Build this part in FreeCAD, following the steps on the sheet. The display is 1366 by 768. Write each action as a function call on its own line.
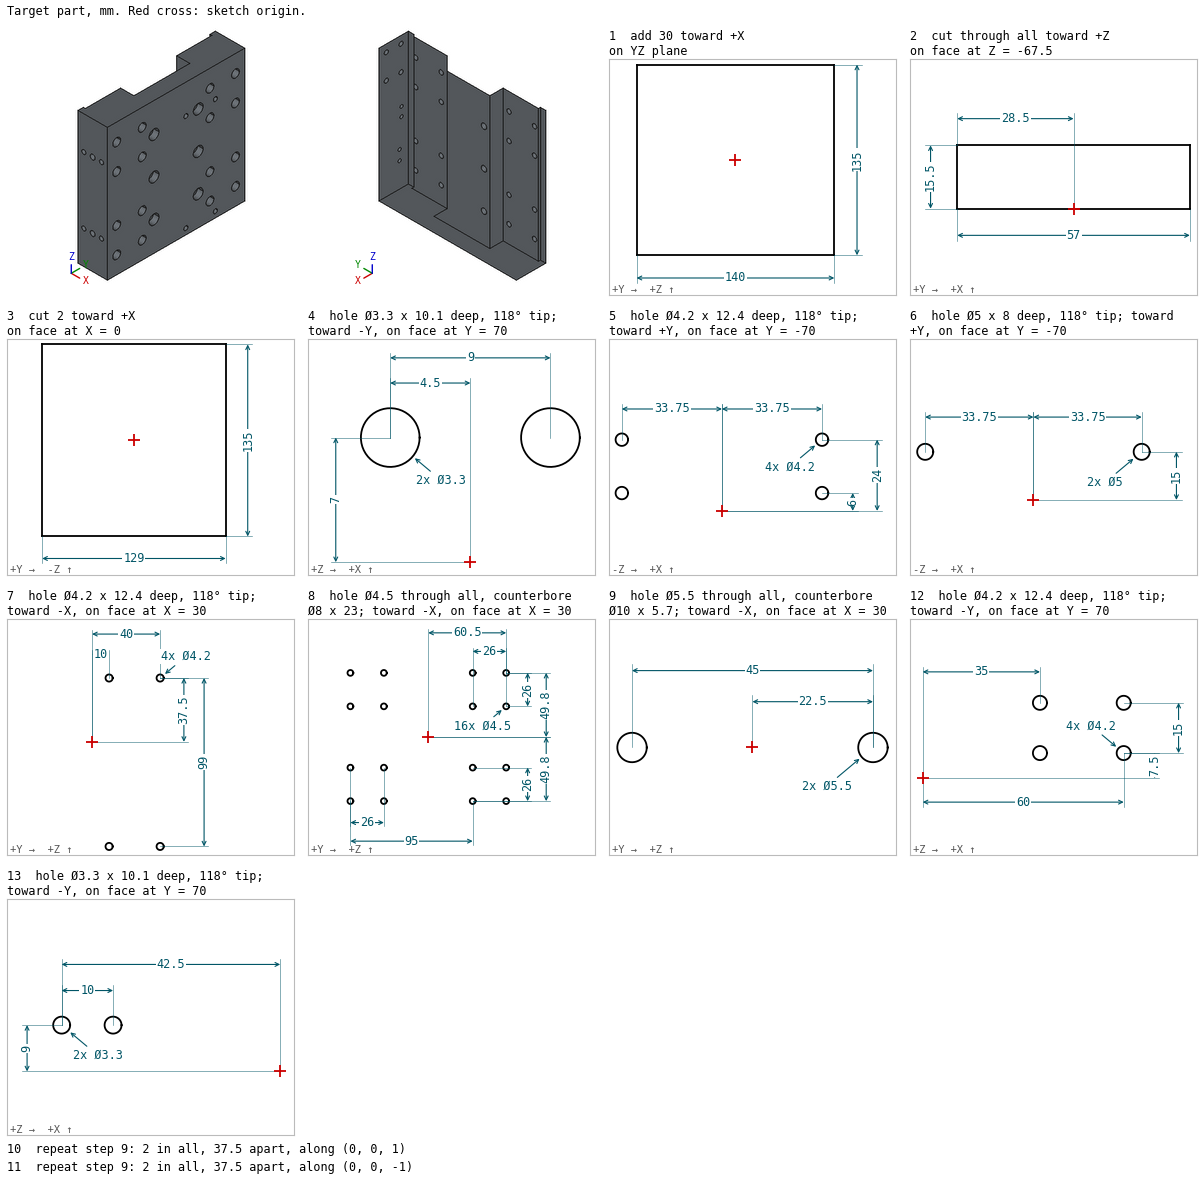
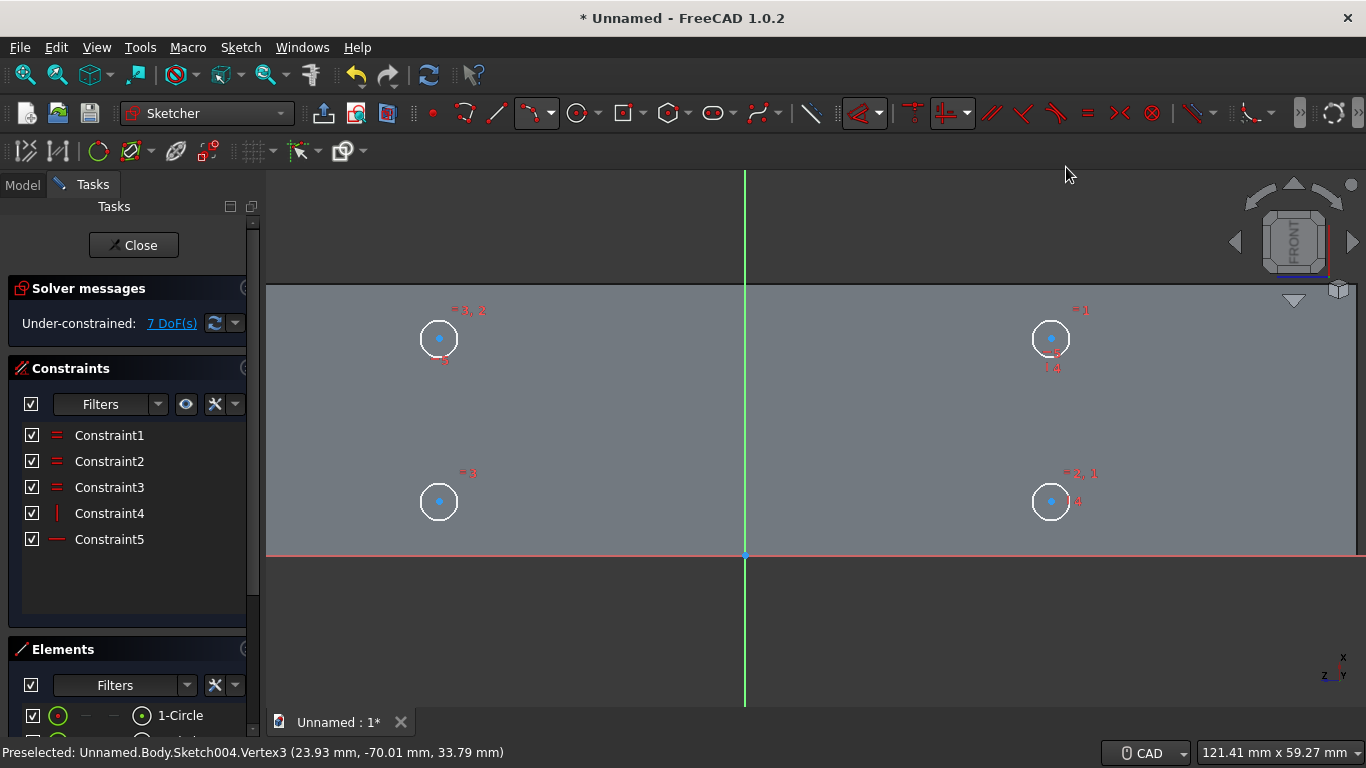
click(439, 339)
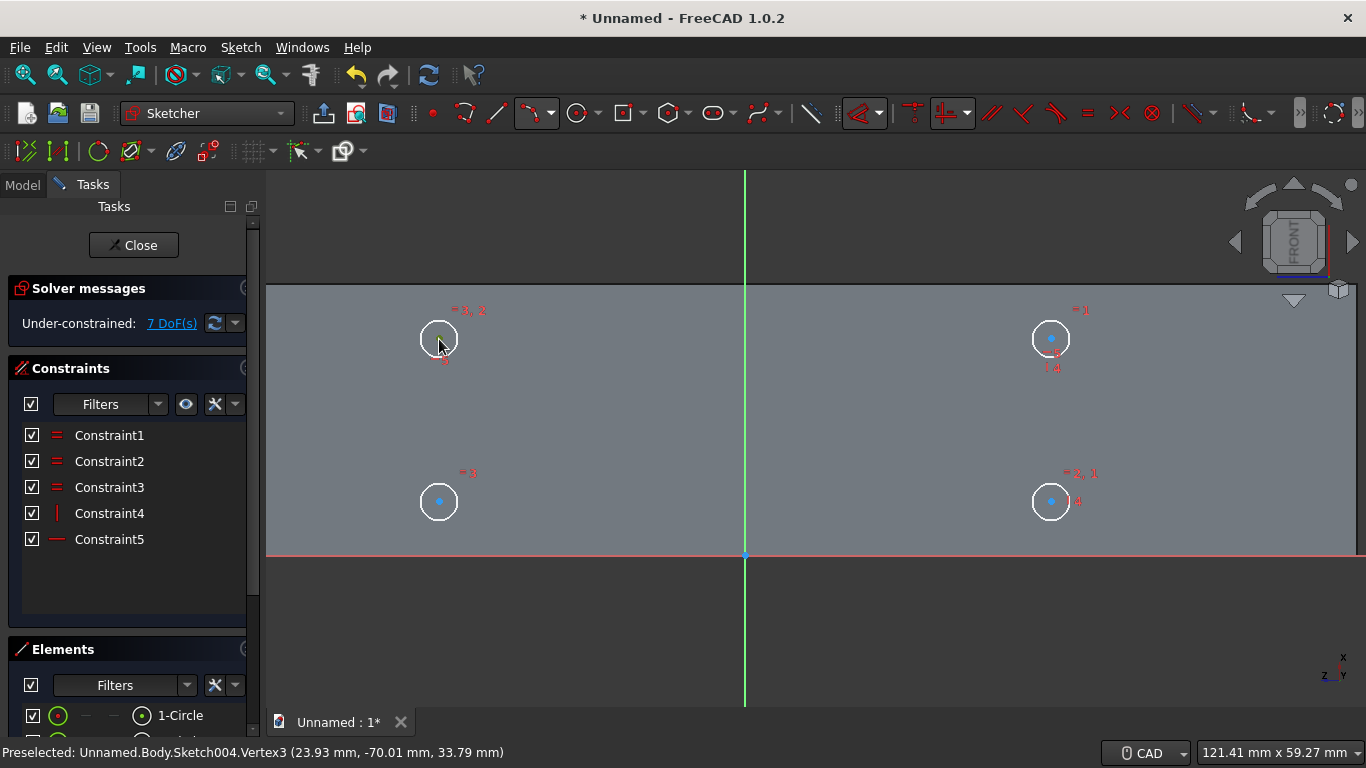
click(439, 502)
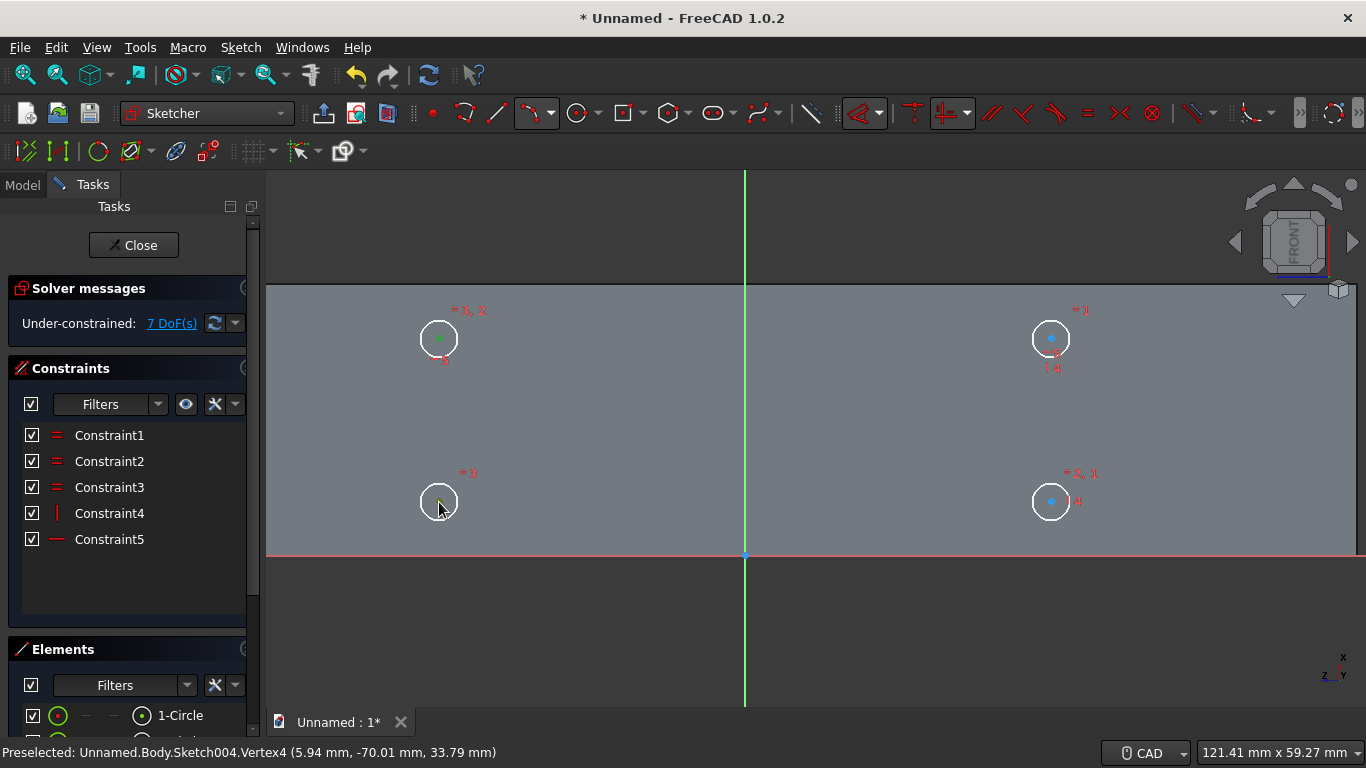
click(970, 114)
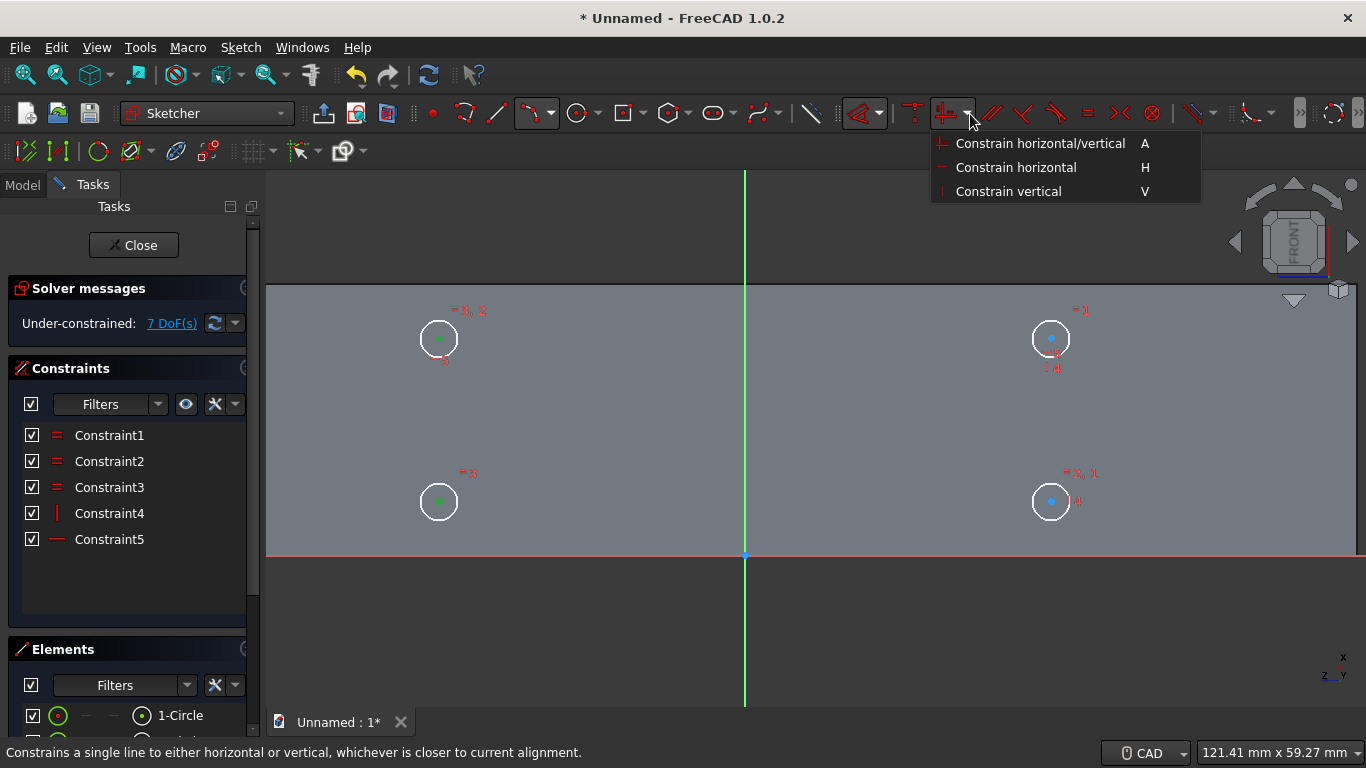
click(1066, 191)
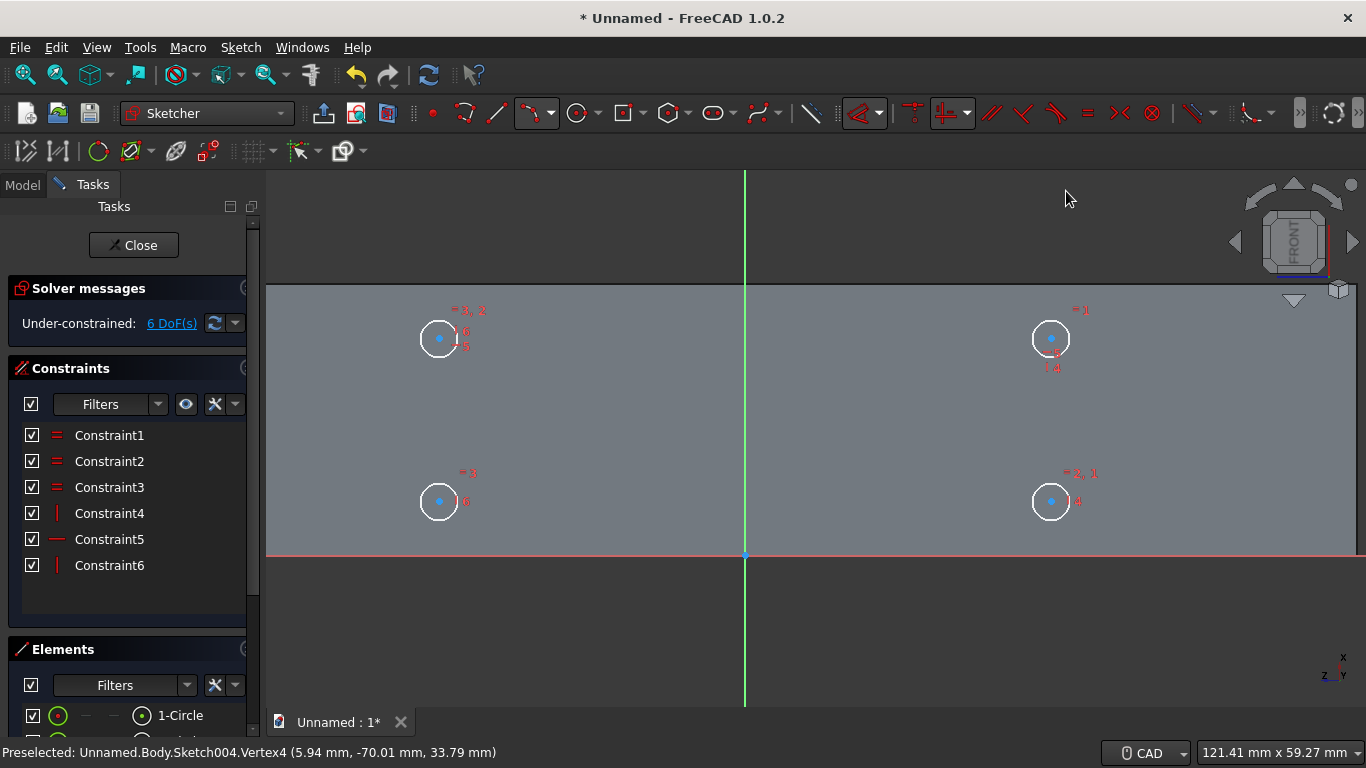
click(1051, 502)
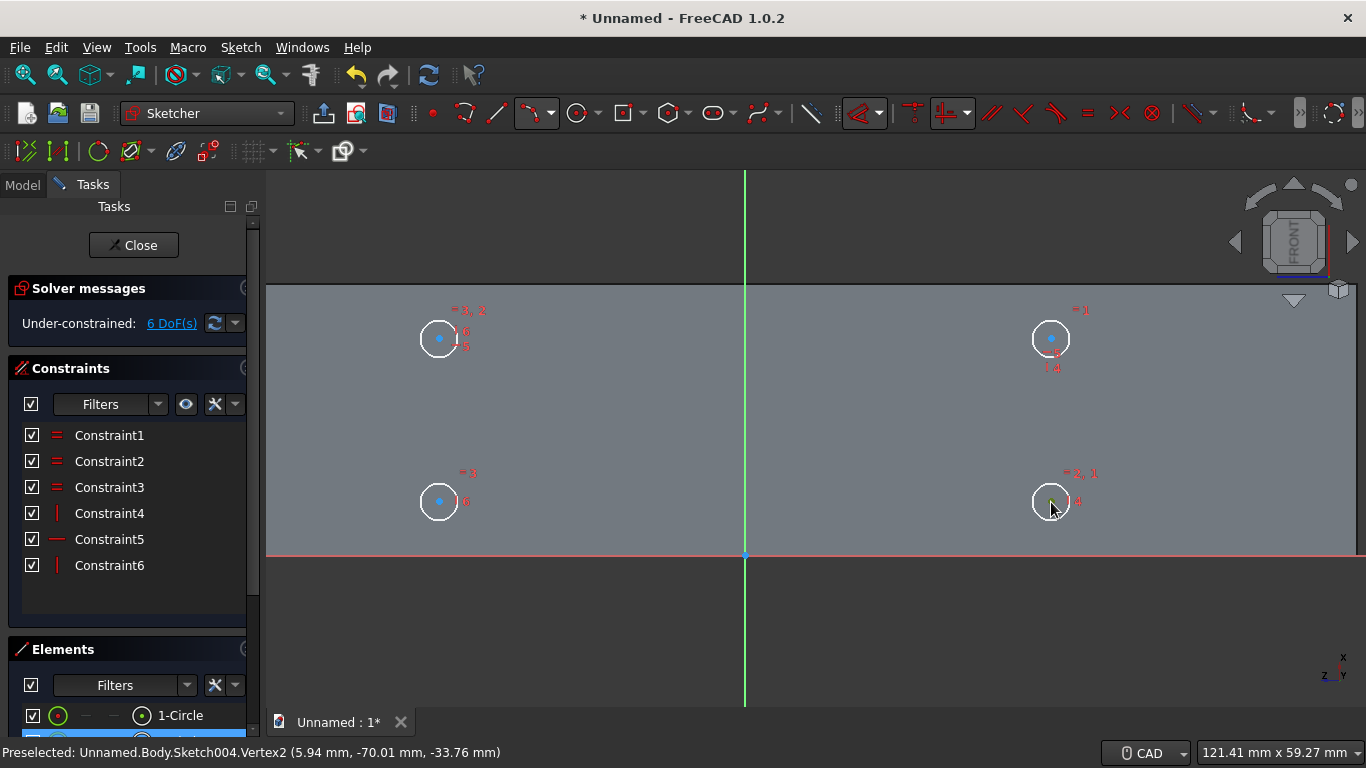
click(439, 502)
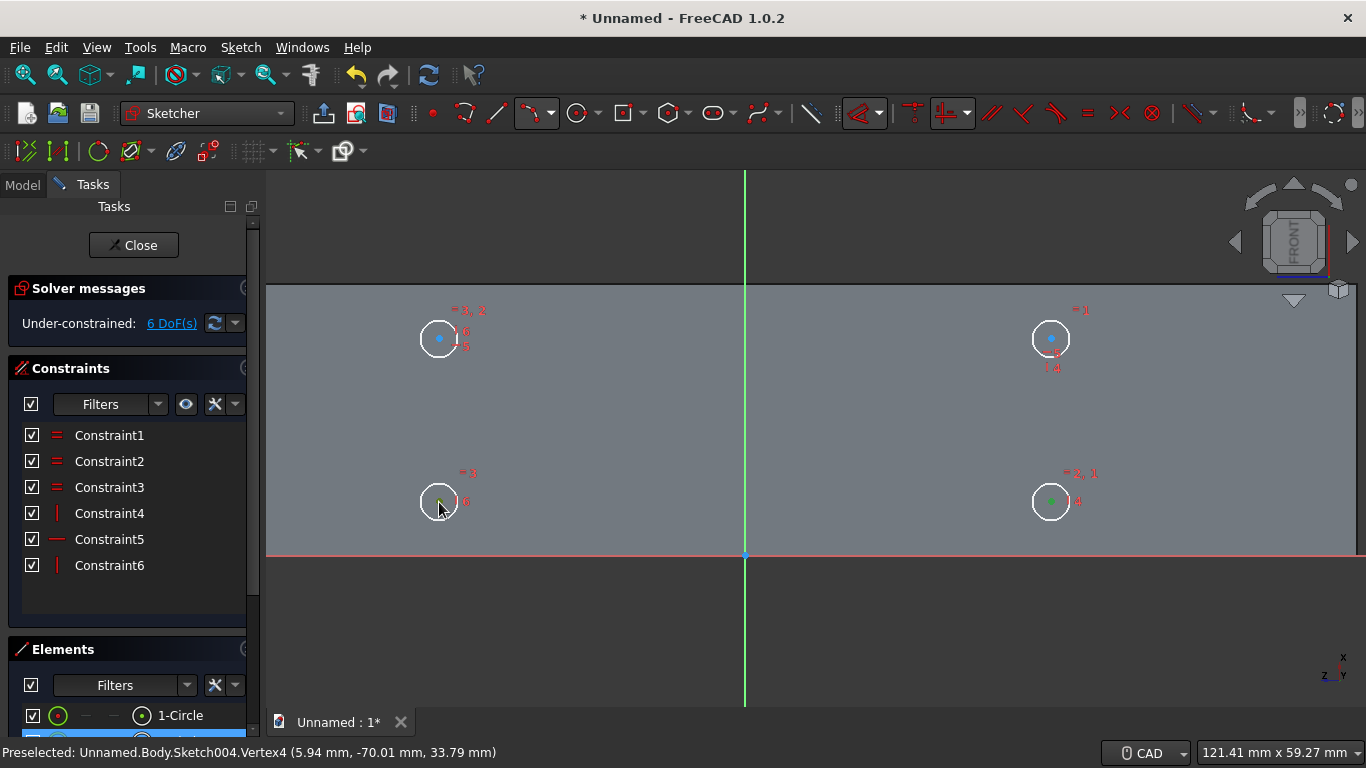
key(h)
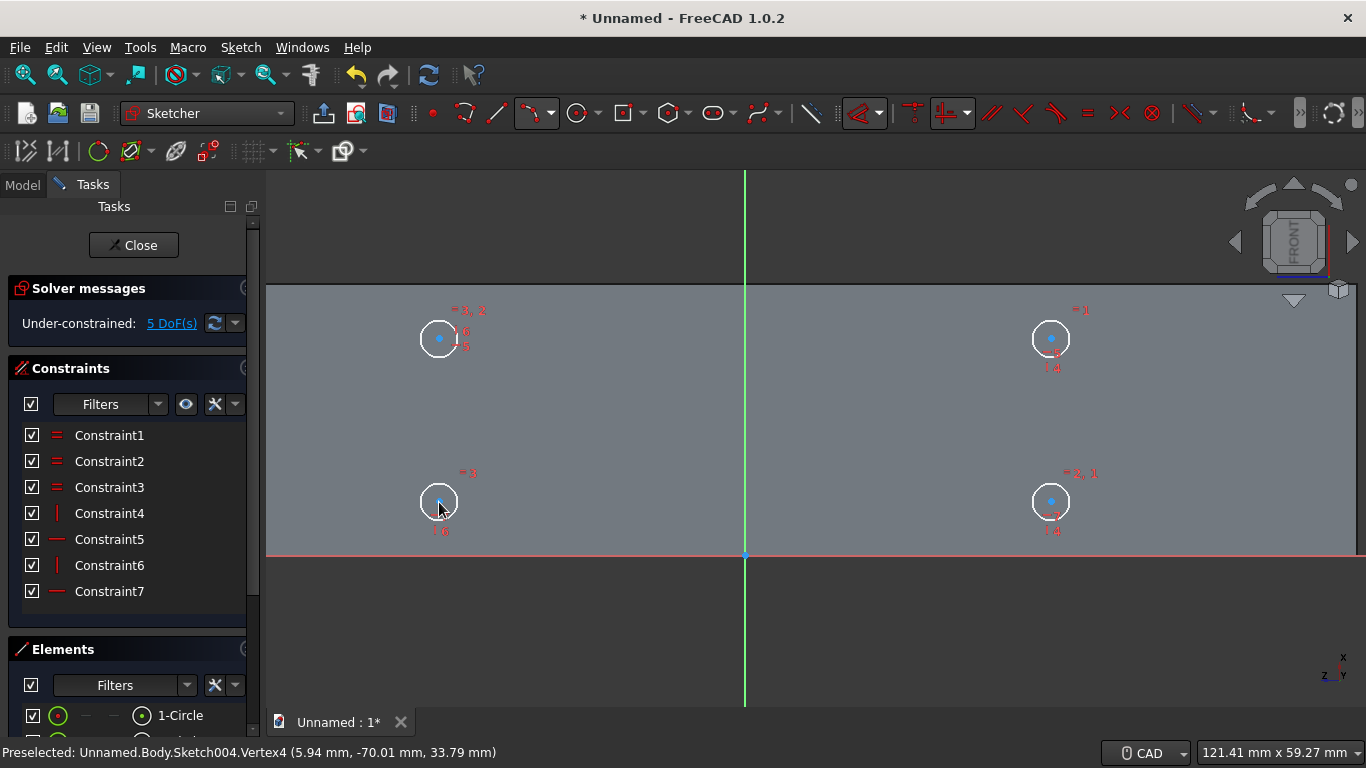
click(1064, 326)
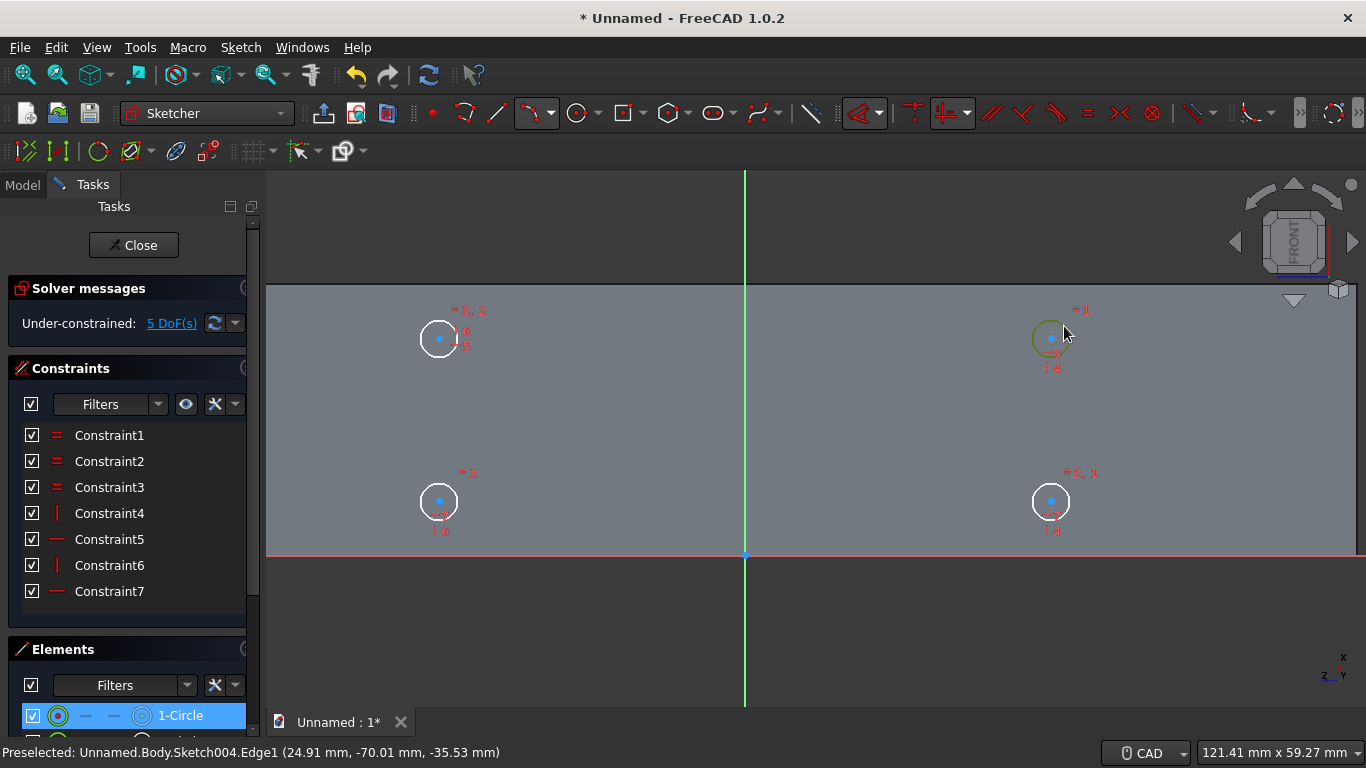
key(k)
key(o)